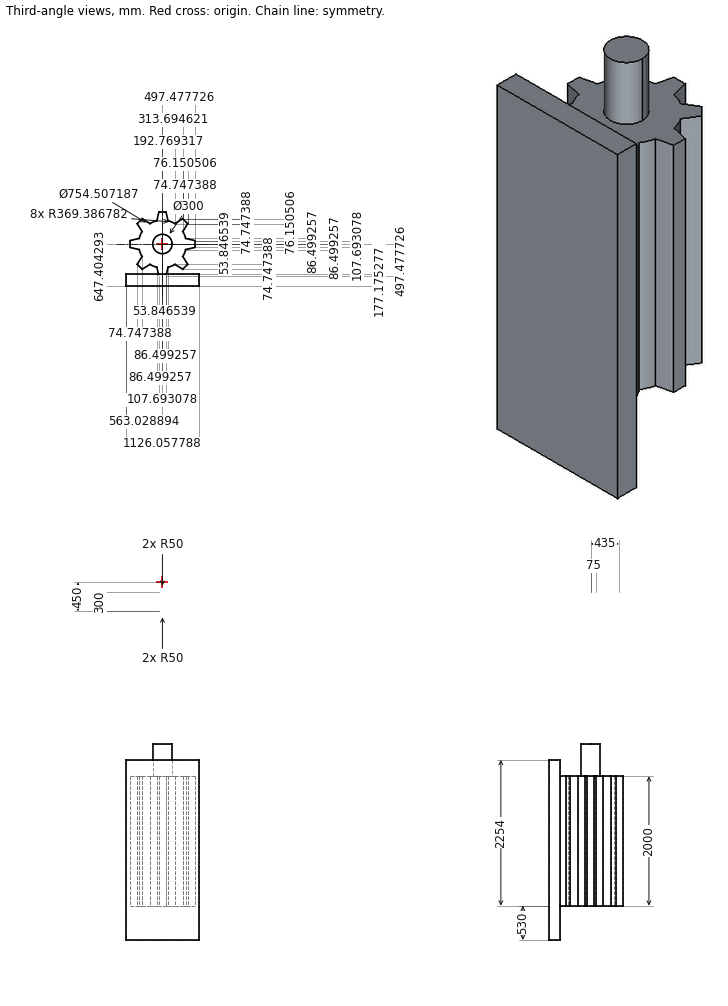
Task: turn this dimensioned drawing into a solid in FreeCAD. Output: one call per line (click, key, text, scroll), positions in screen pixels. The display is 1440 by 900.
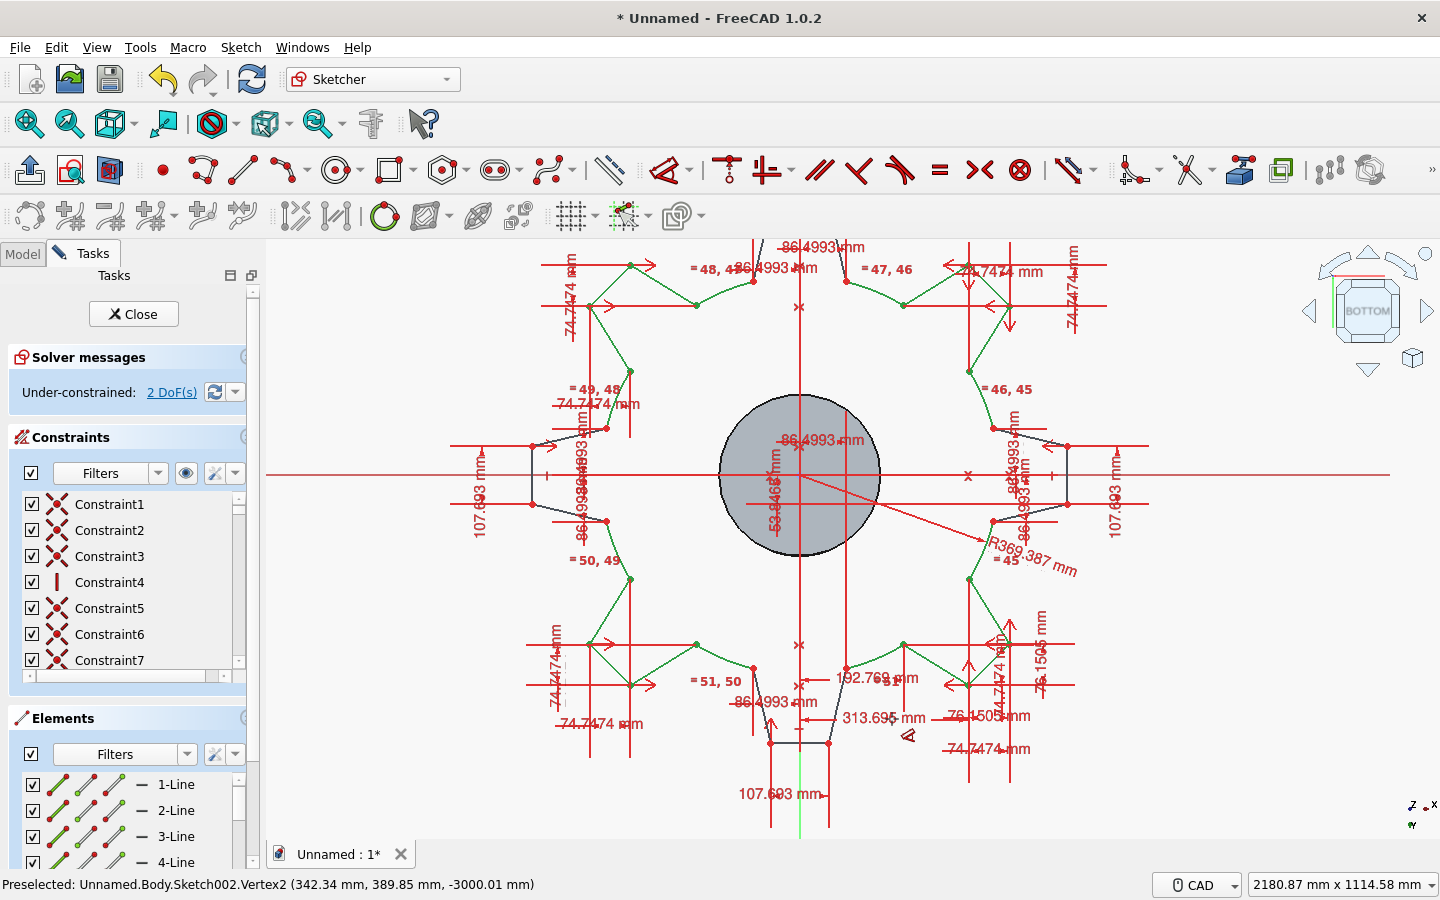
click(1067, 504)
click(934, 538)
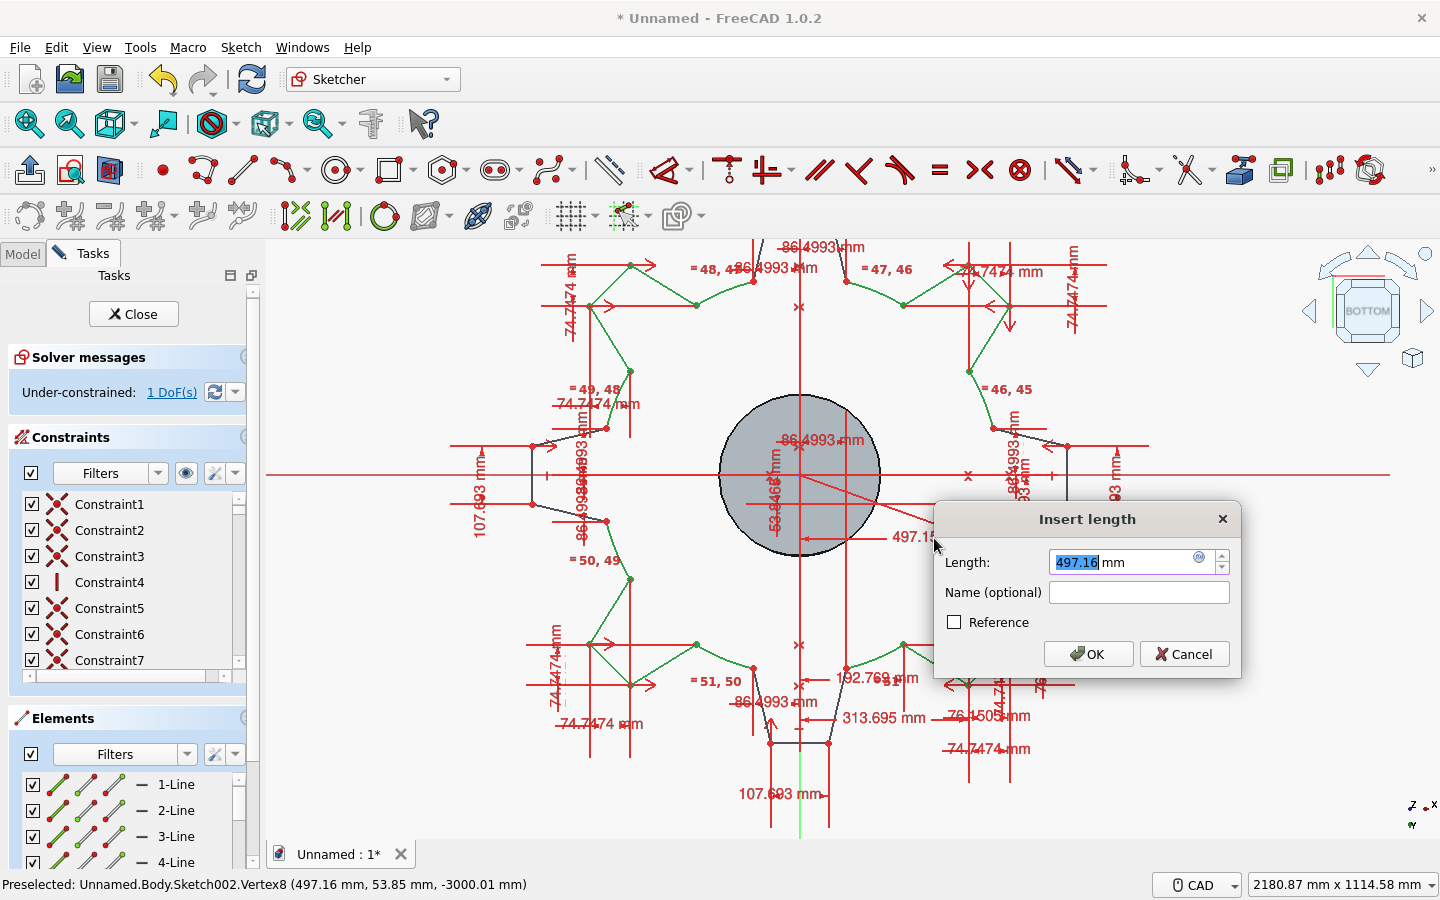
text(497.477726)
key(Return)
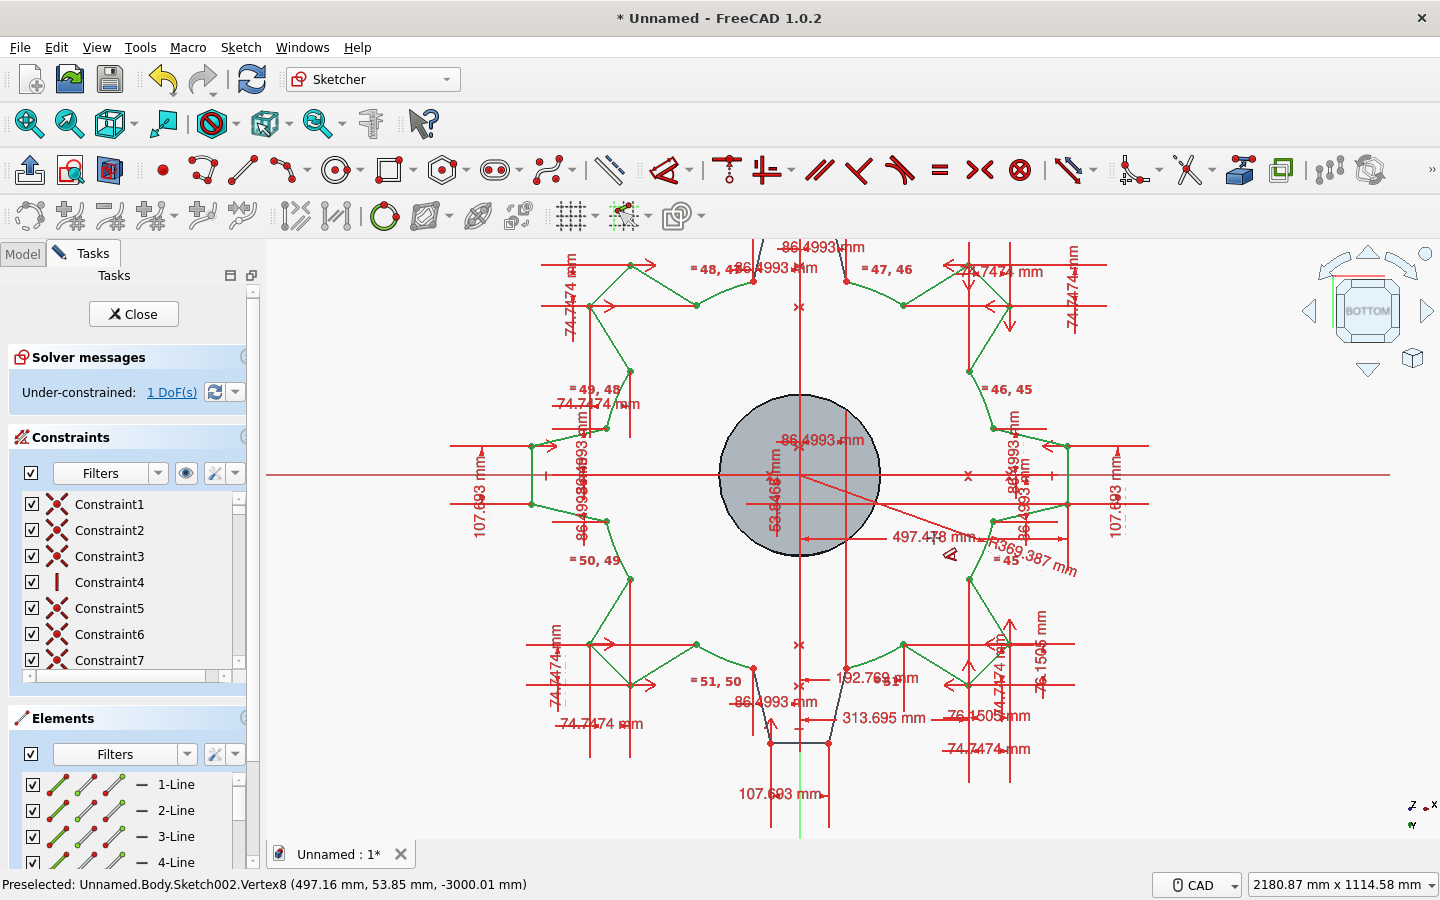
scroll(753, 669, down, 2)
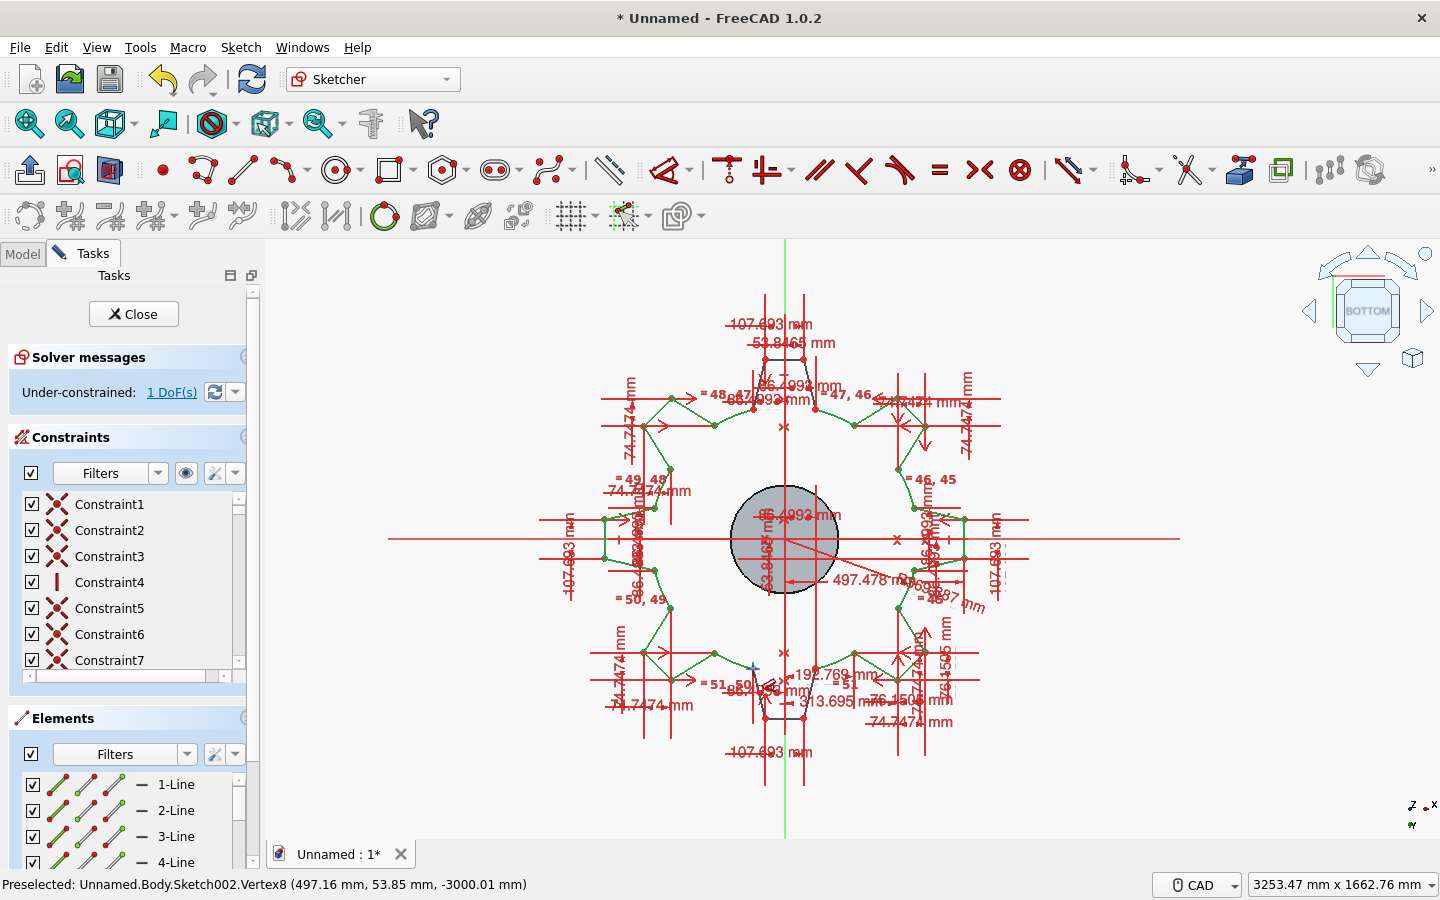
click(804, 360)
click(838, 450)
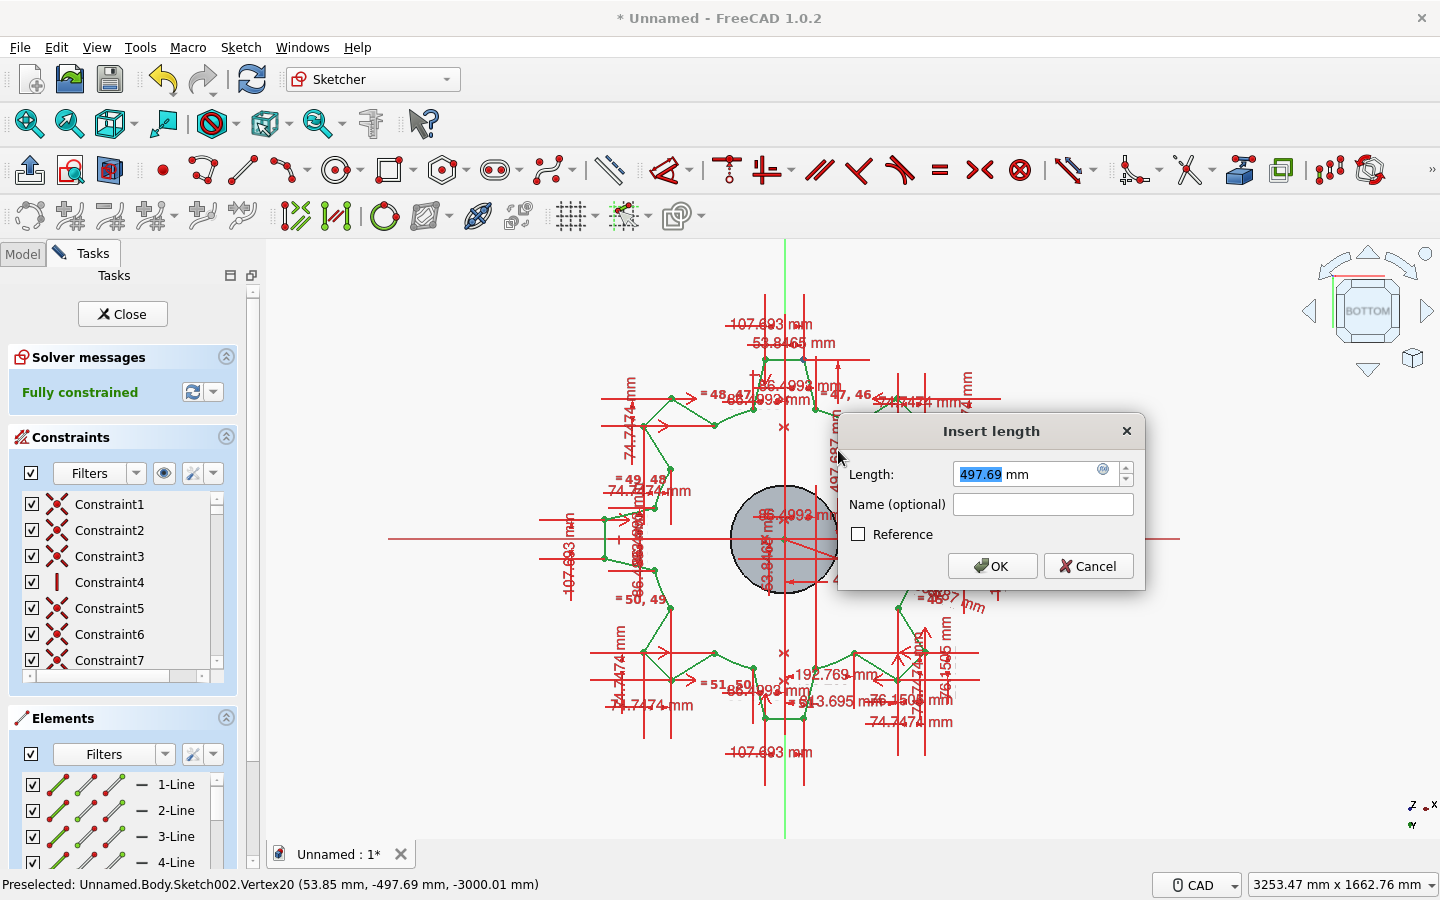
text(497.477726)
key(Return)
key(Escape)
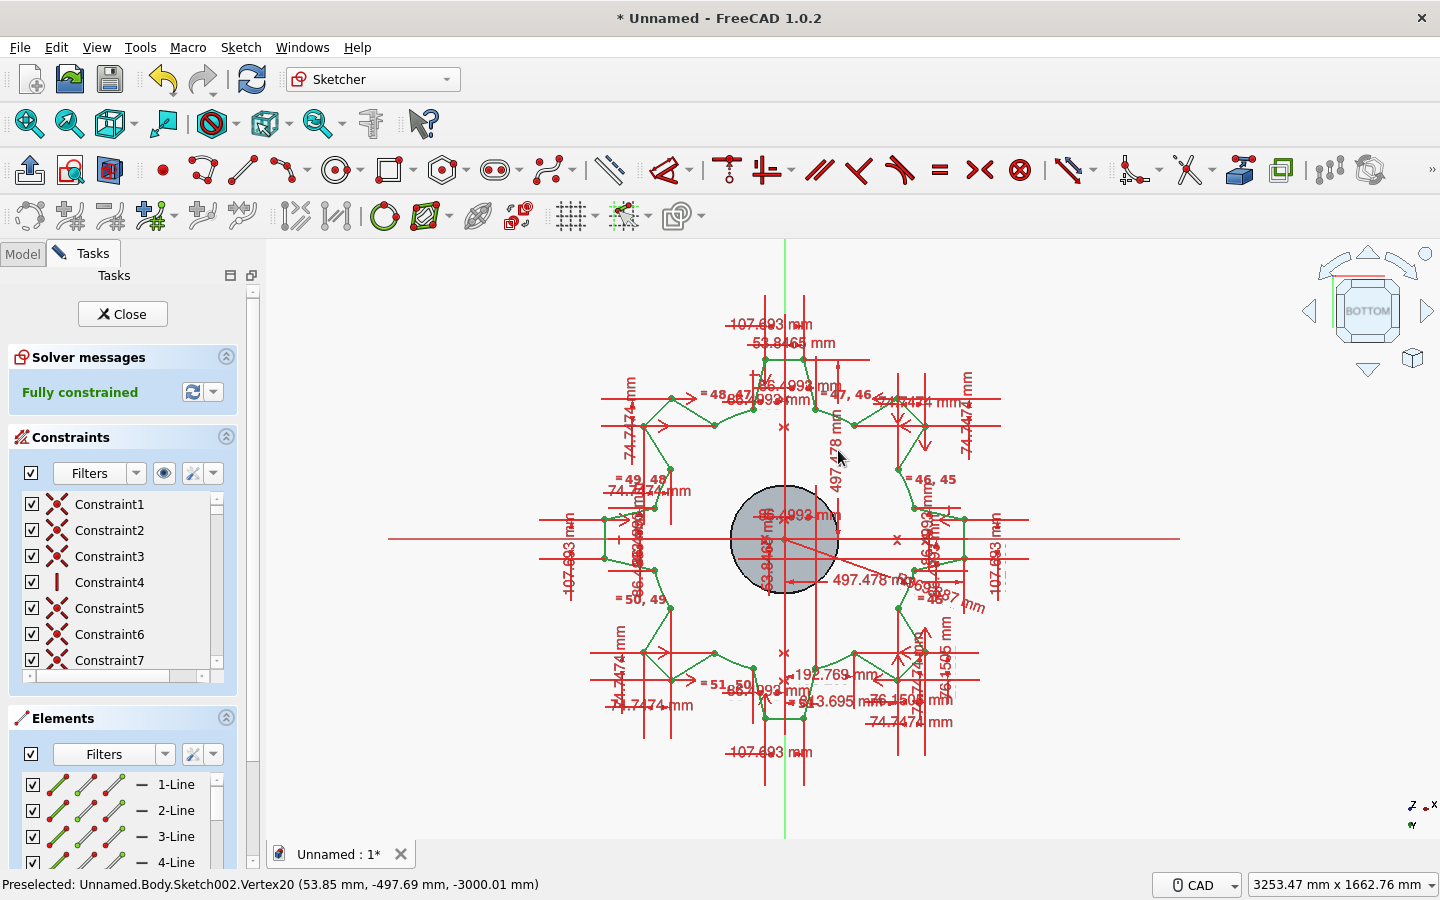
click(123, 314)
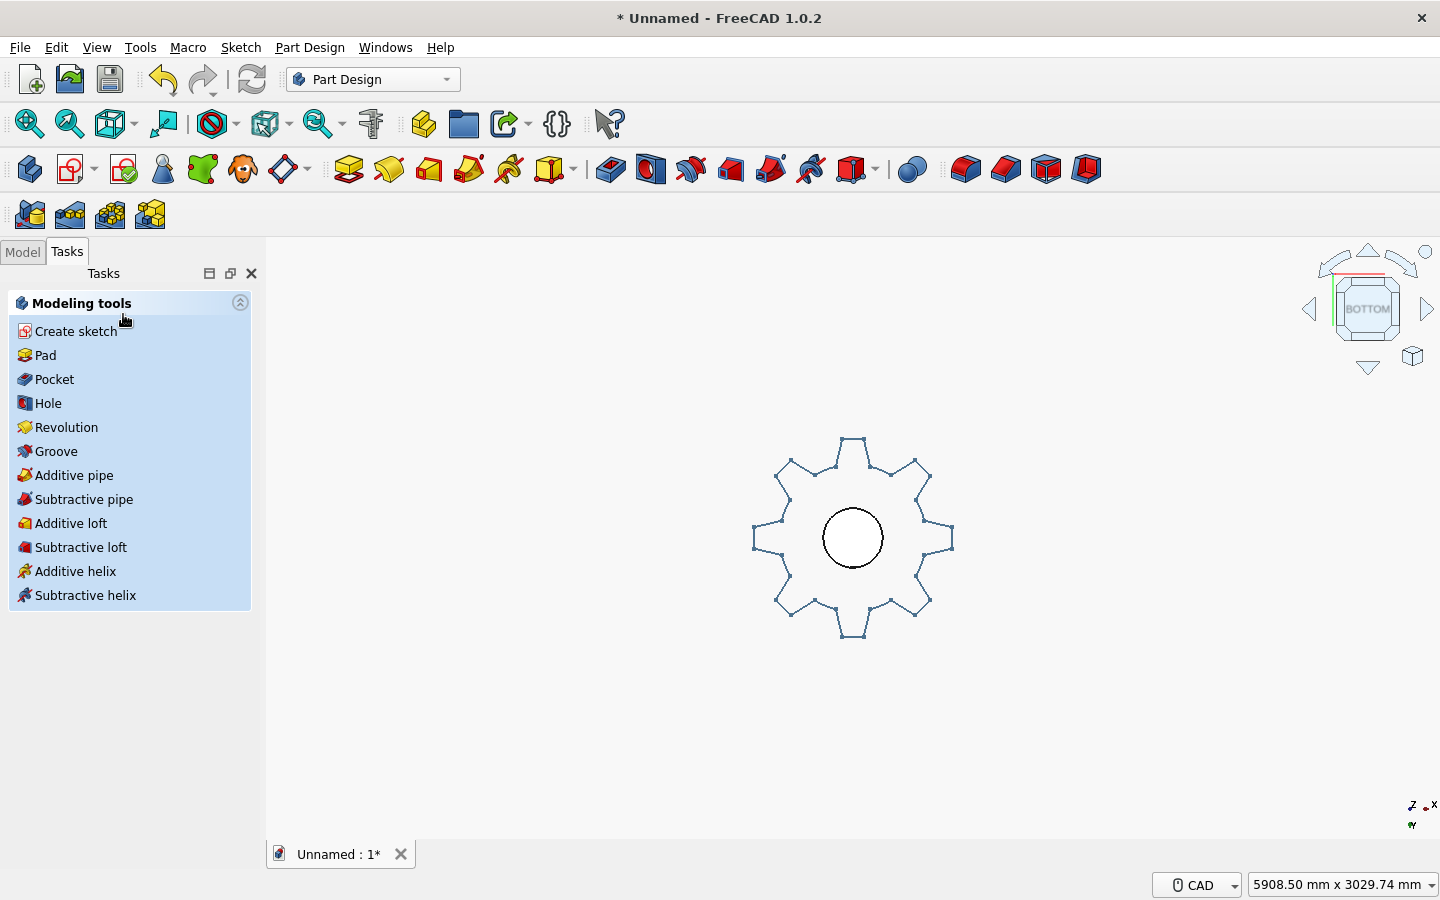
click(350, 170)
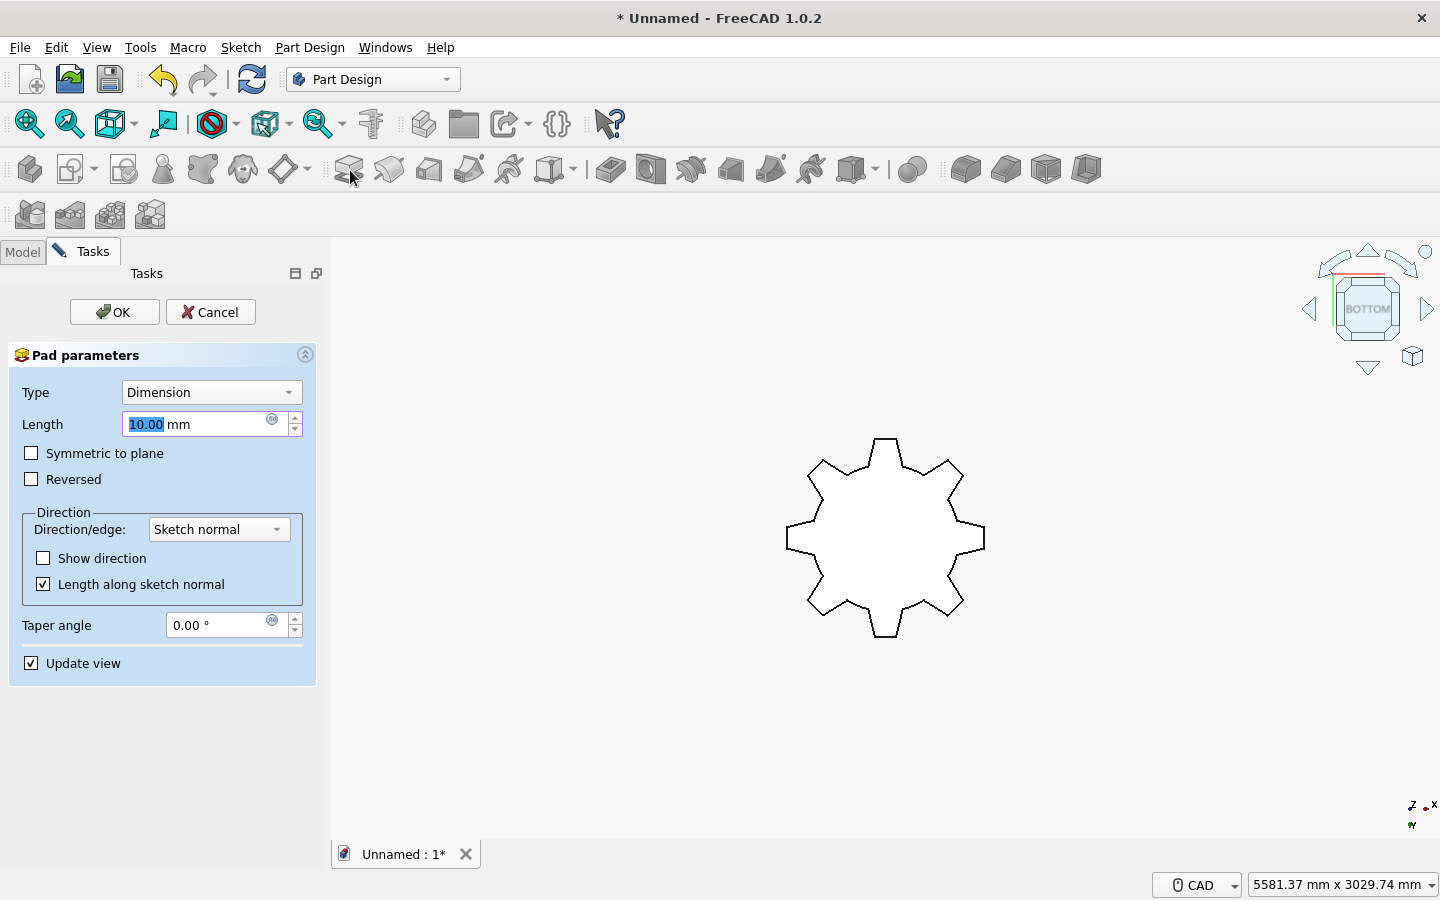
text(2000)
key(Tab)